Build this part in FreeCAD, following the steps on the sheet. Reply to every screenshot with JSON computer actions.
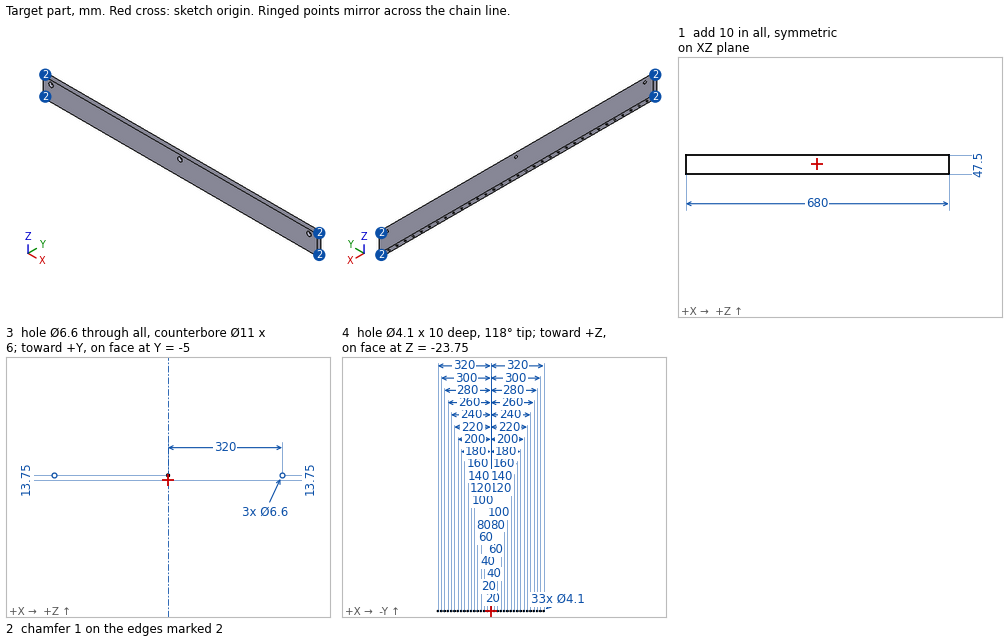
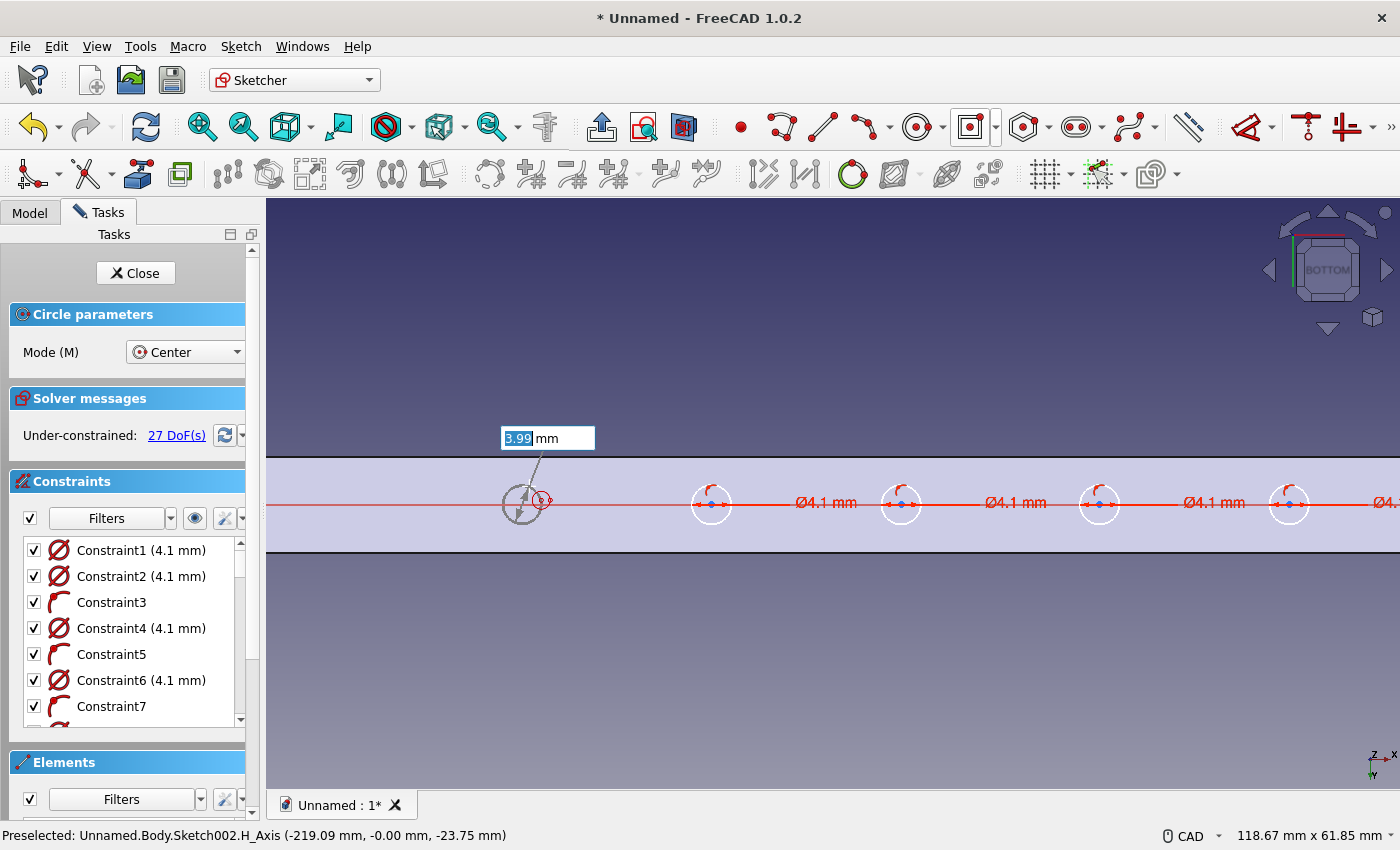
{"action": "type", "text": "4.1"}
{"action": "key", "text": "Return"}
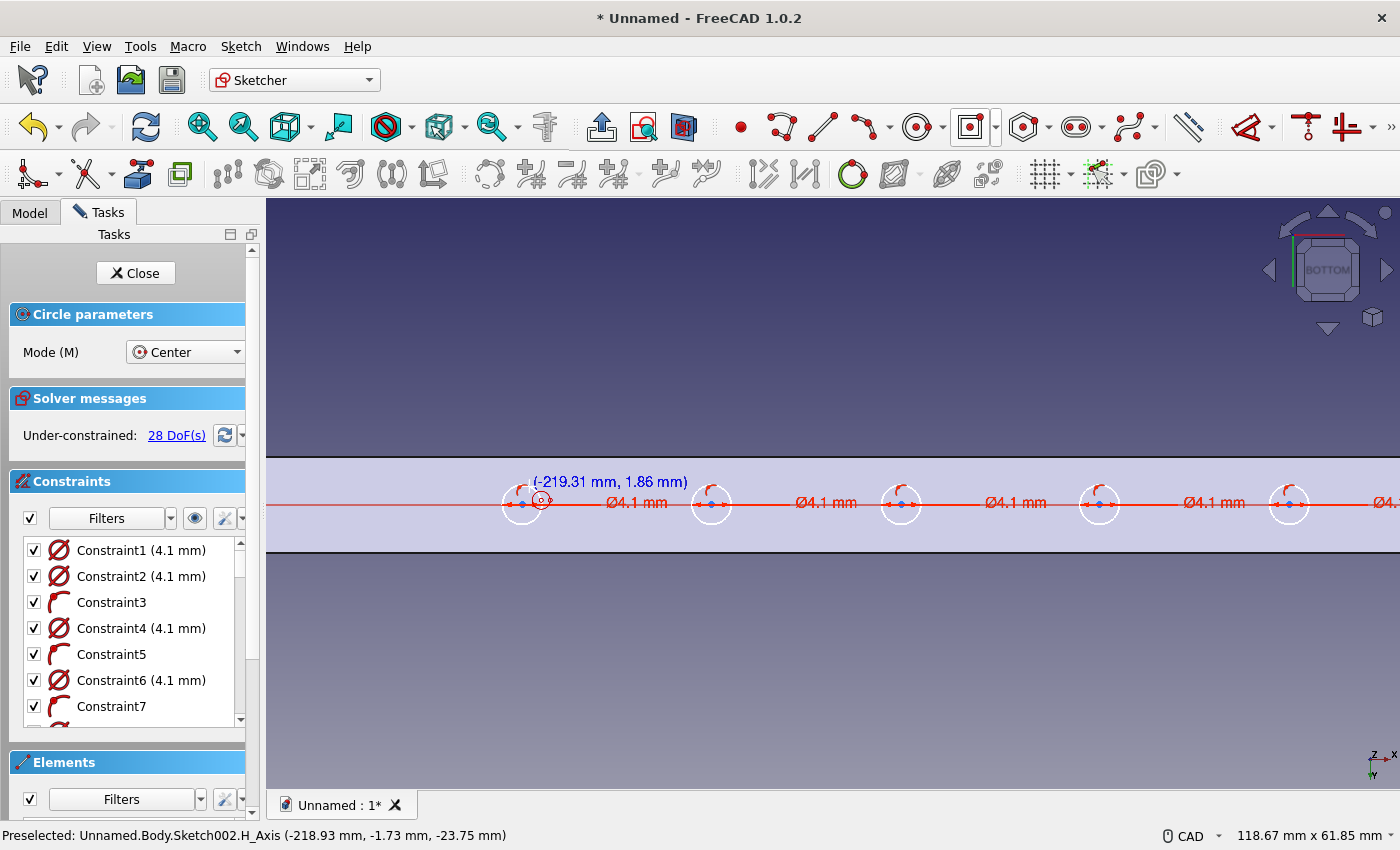
{"action": "scroll", "coordinate": [533, 492], "scroll_direction": "down", "scroll_amount": 11}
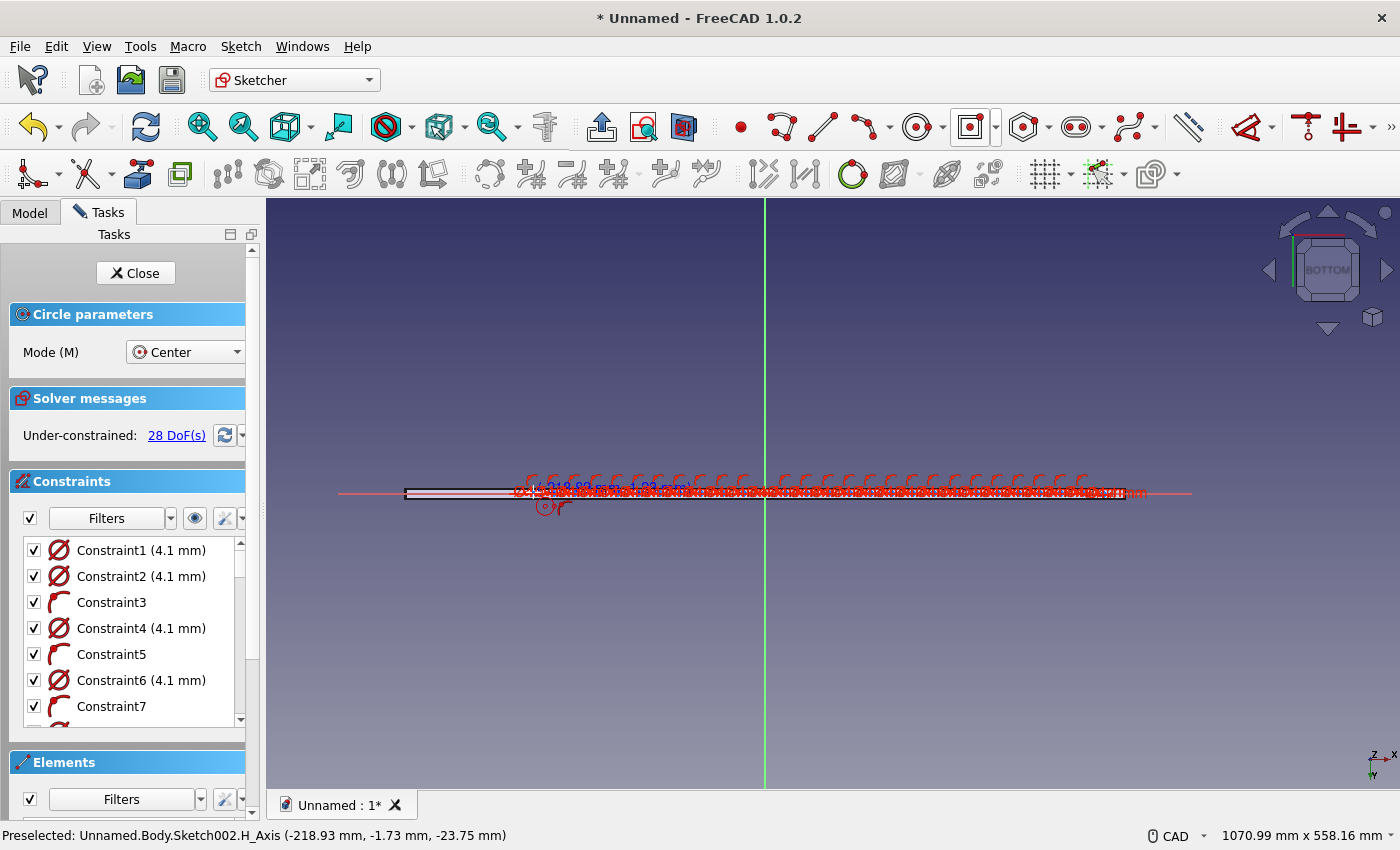
{"action": "left_click", "coordinate": [511, 494]}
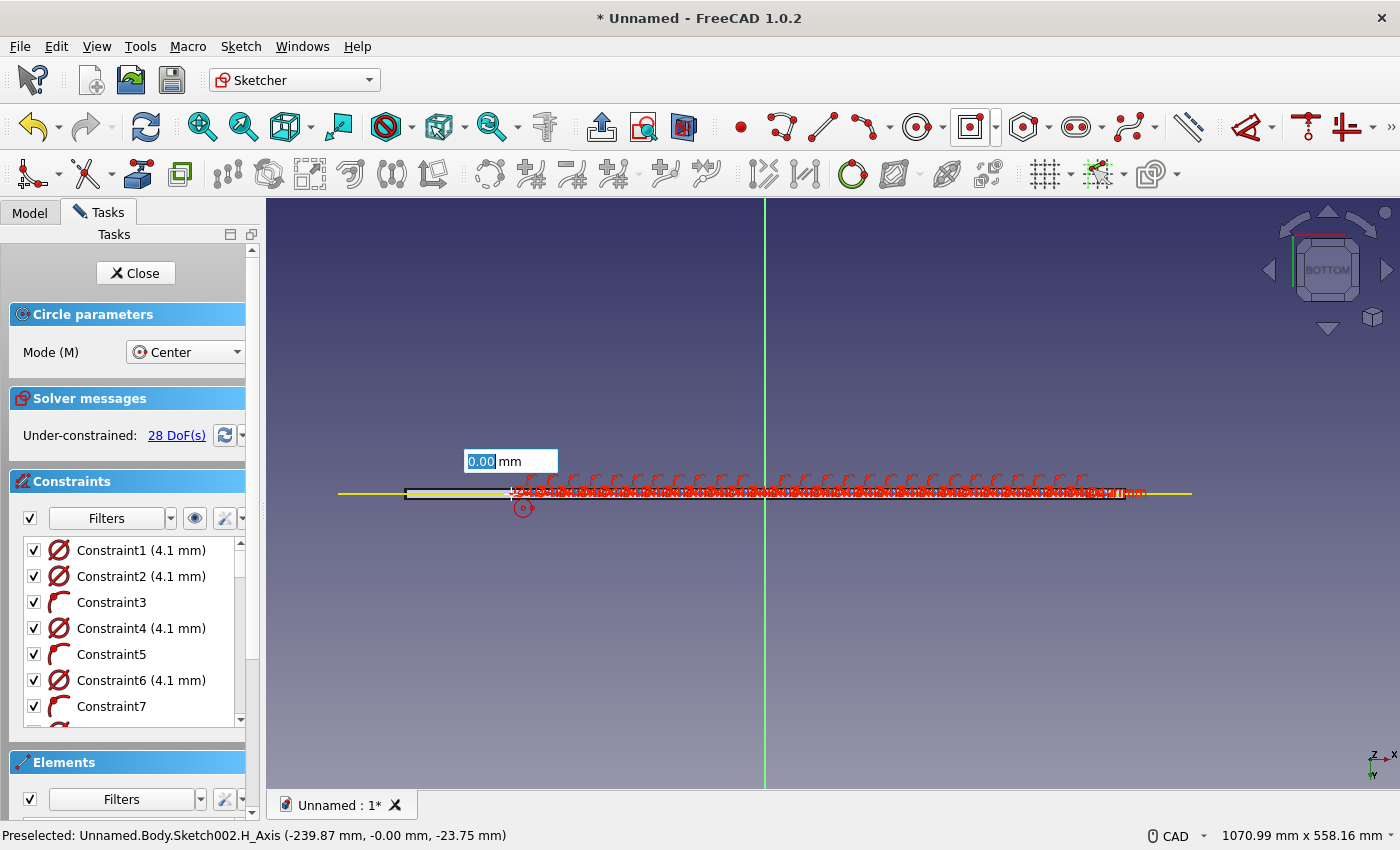
{"action": "scroll", "coordinate": [510, 496], "scroll_direction": "up", "scroll_amount": 11}
{"action": "mouse_move", "coordinate": [509, 491]}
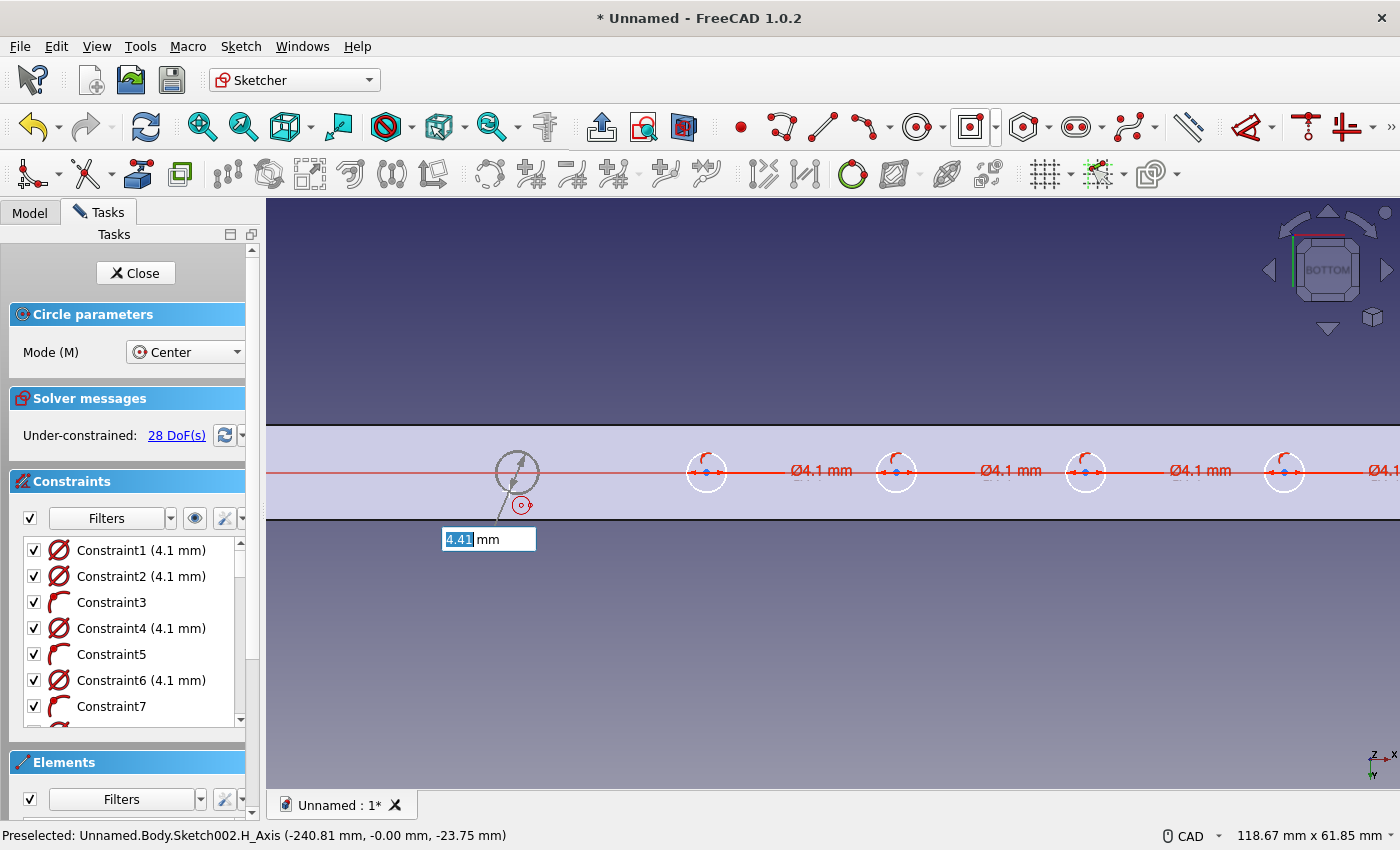
{"action": "type", "text": "4.1"}
{"action": "key", "text": "Return"}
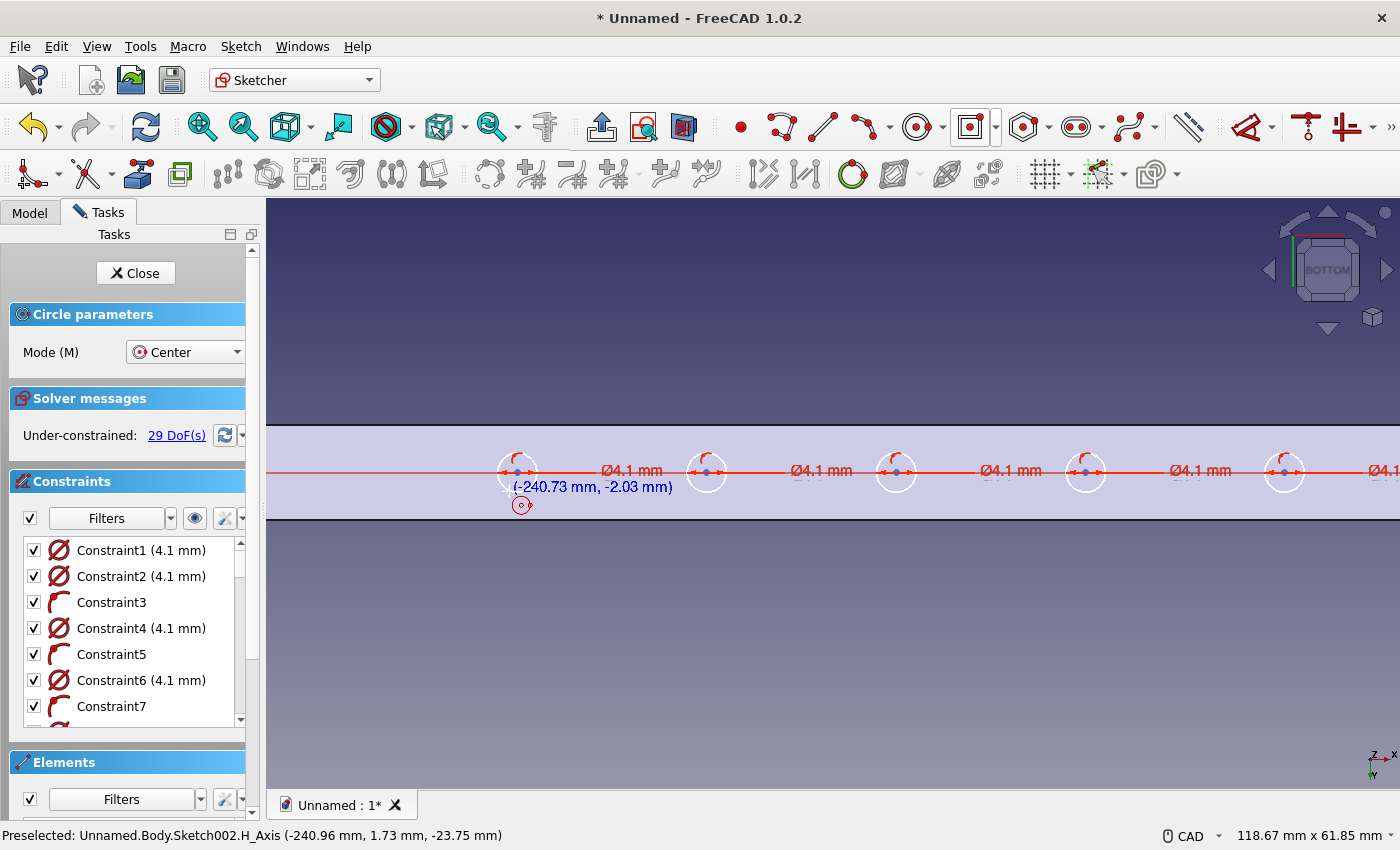
{"action": "scroll", "coordinate": [510, 496], "scroll_direction": "down", "scroll_amount": 11}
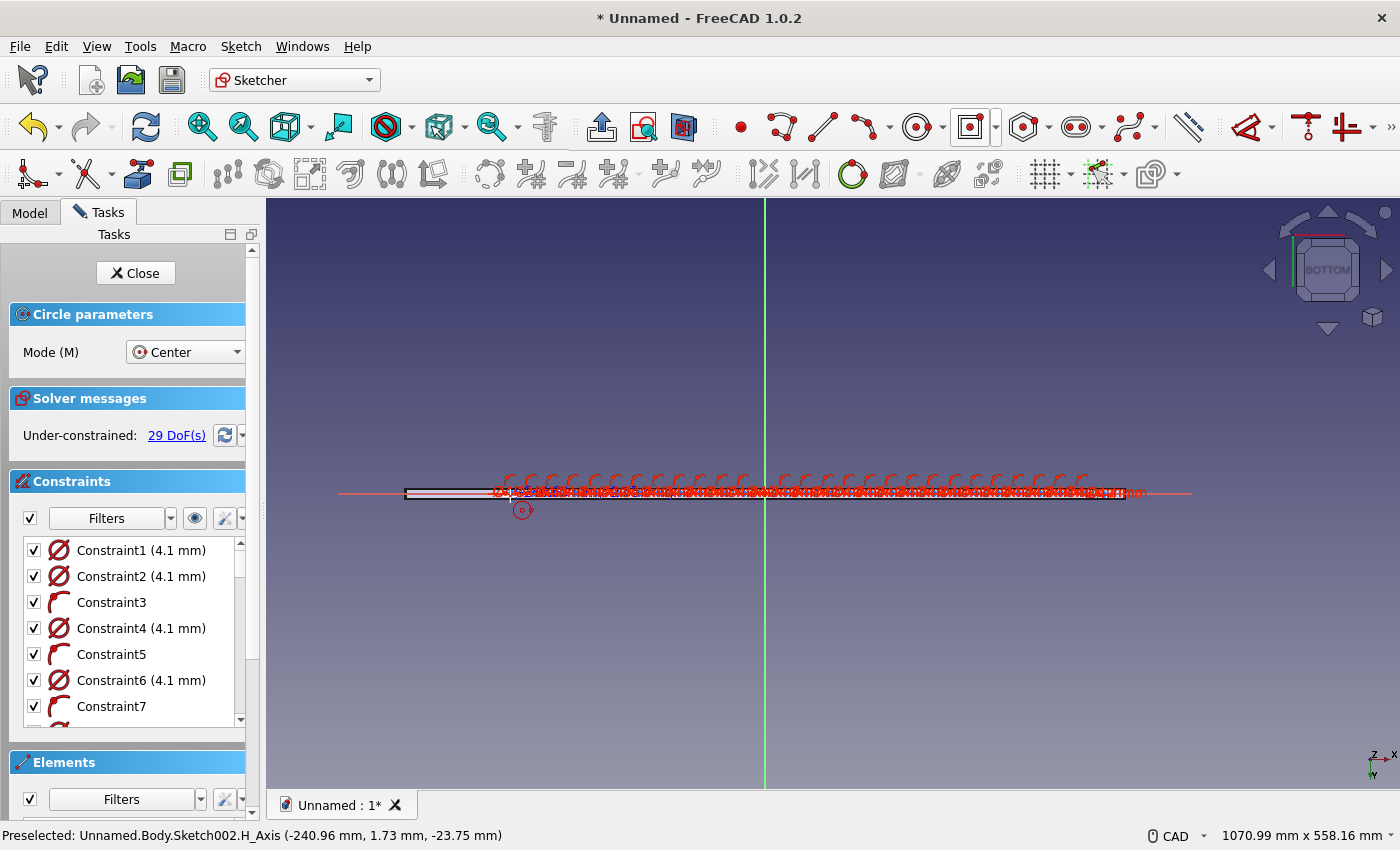
{"action": "left_click", "coordinate": [490, 494]}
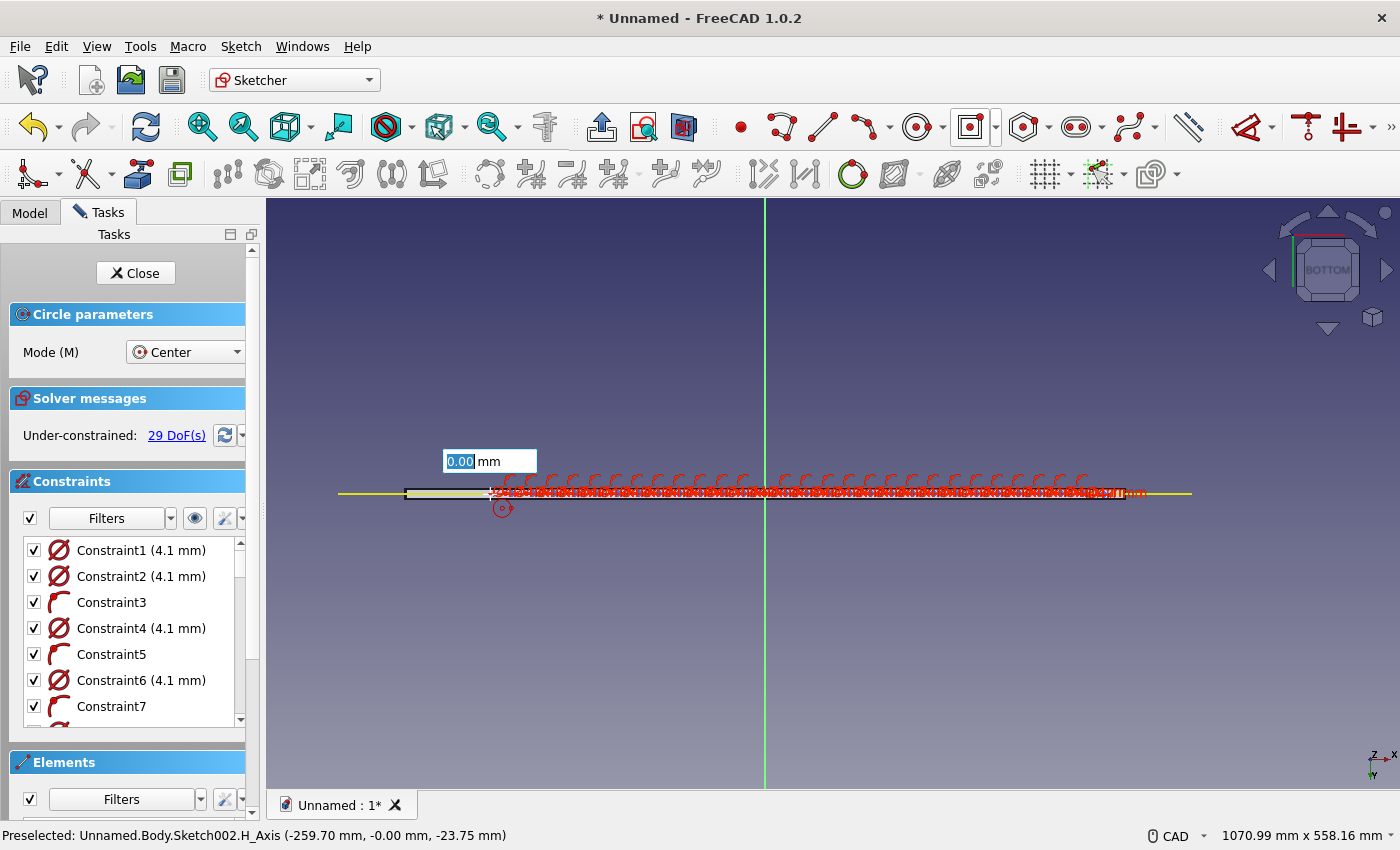
{"action": "scroll", "coordinate": [490, 492], "scroll_direction": "up", "scroll_amount": 11}
{"action": "mouse_move", "coordinate": [492, 486]}